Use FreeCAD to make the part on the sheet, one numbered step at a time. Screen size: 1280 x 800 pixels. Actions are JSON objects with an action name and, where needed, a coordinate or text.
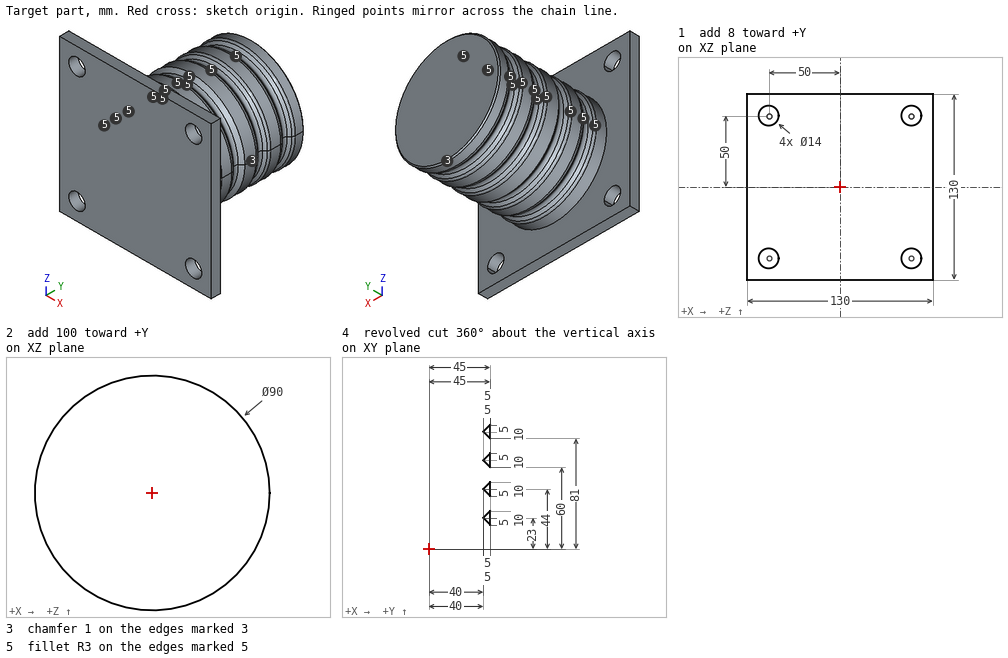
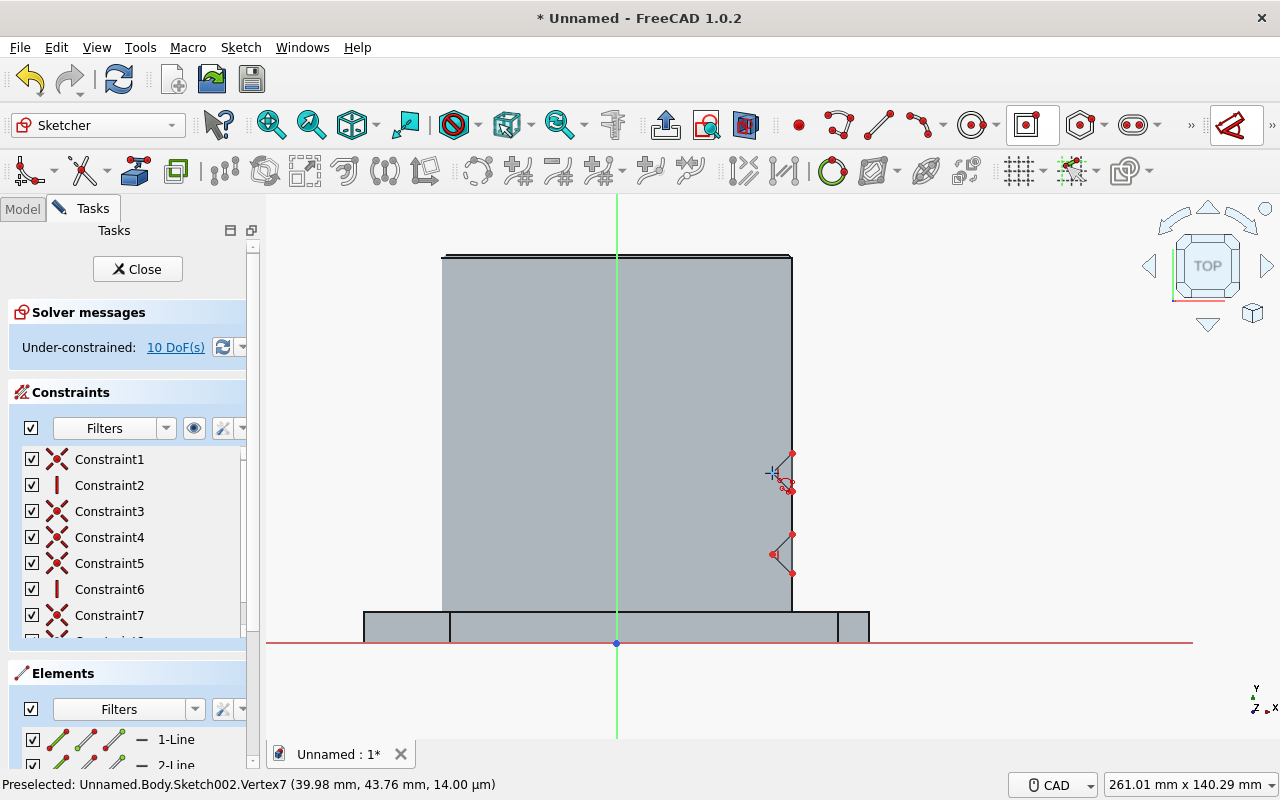
{"action": "left_click", "coordinate": [792, 410]}
{"action": "left_click", "coordinate": [792, 371]}
{"action": "left_click", "coordinate": [772, 390]}
{"action": "left_click", "coordinate": [792, 411]}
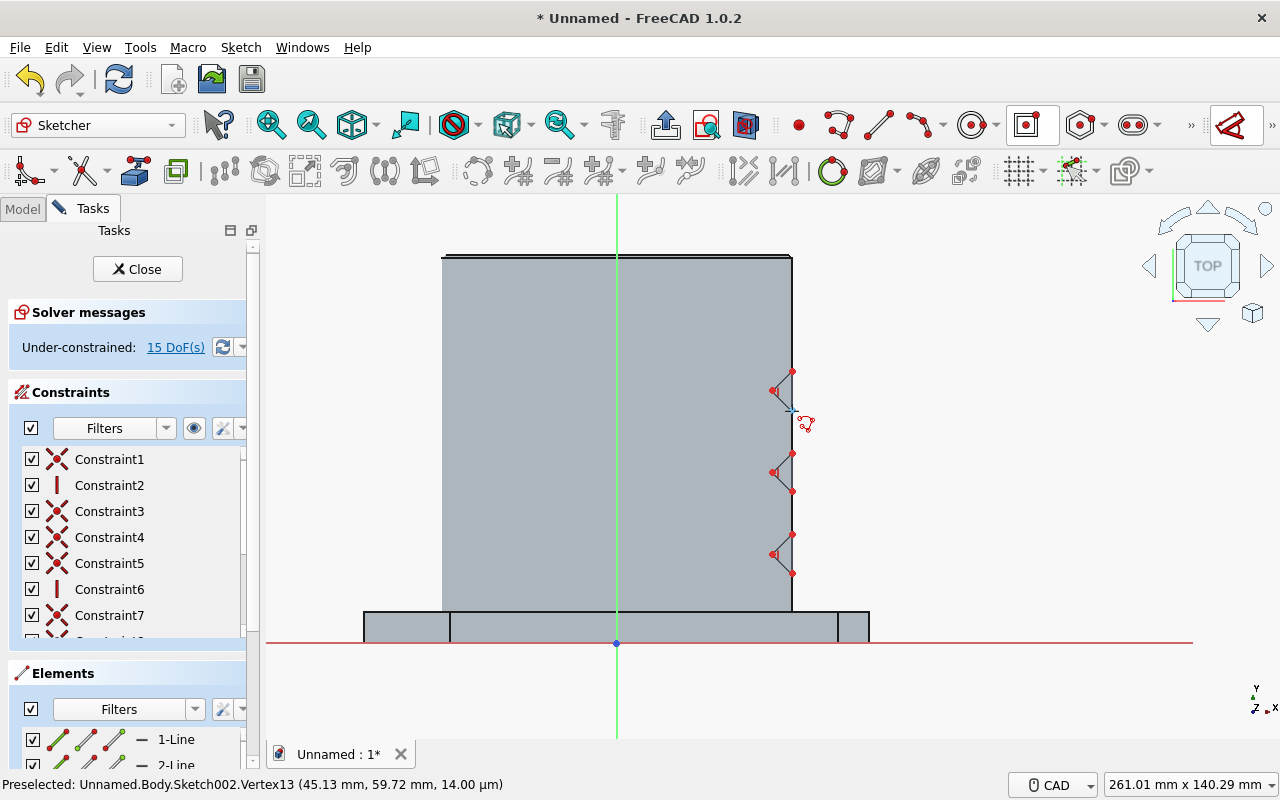
{"action": "left_click", "coordinate": [792, 328]}
{"action": "left_click", "coordinate": [792, 289]}
{"action": "left_click", "coordinate": [772, 309]}
{"action": "left_click", "coordinate": [792, 329]}
{"action": "key", "text": "Escape"}
{"action": "key", "text": "Escape"}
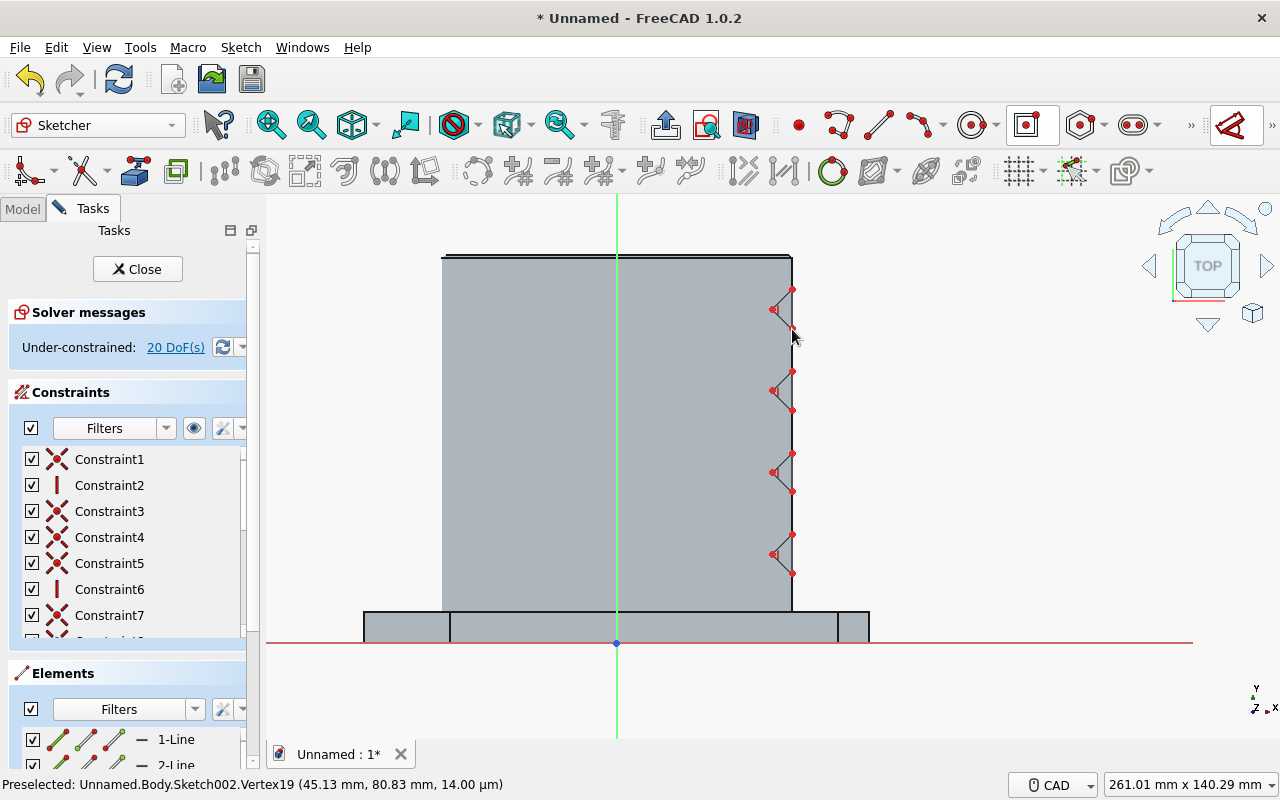
{"action": "left_click", "coordinate": [792, 558]}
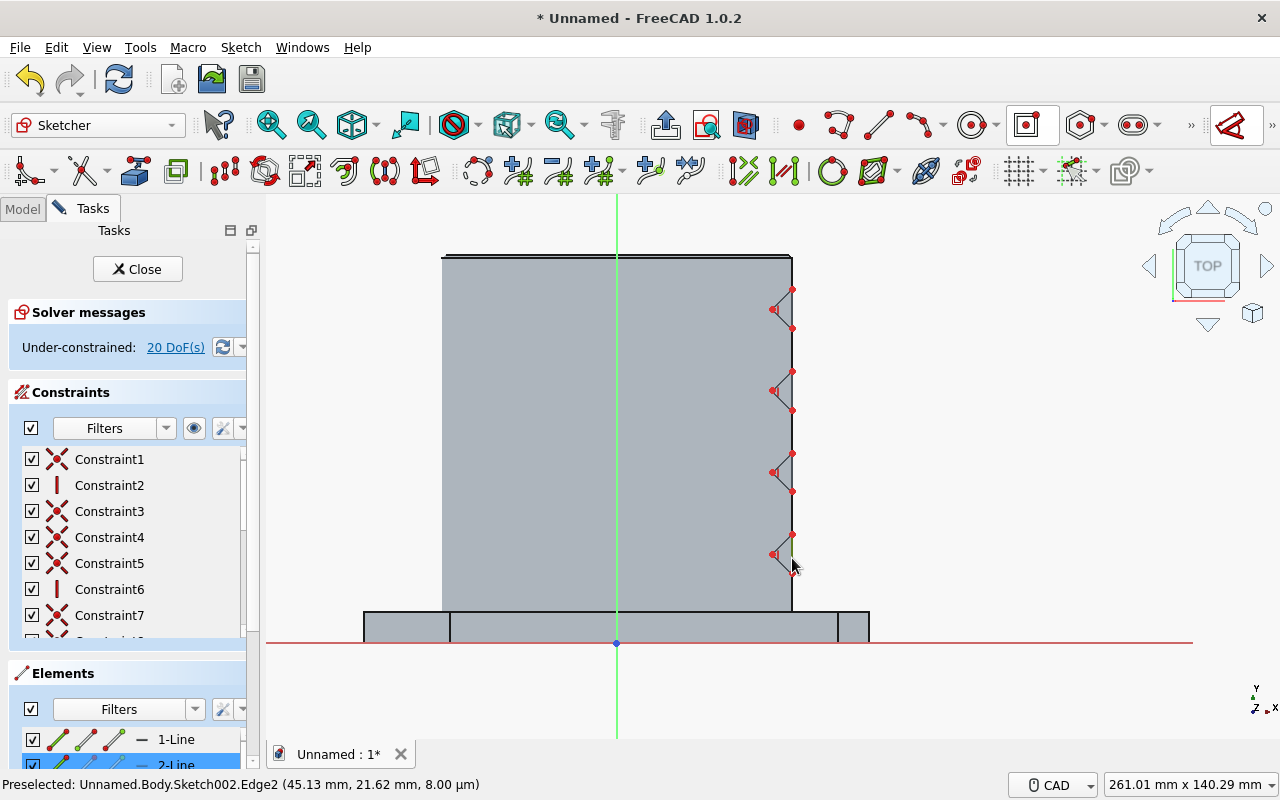
{"action": "key", "text": "i"}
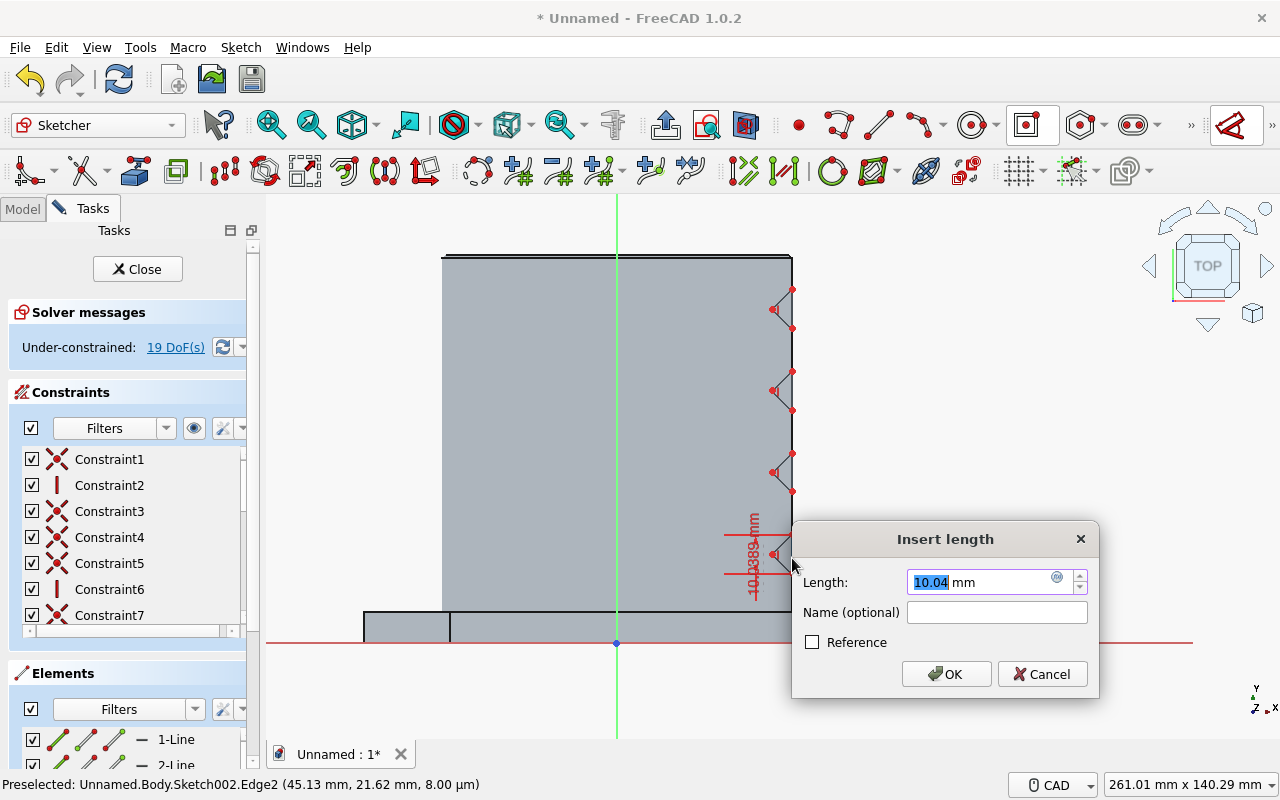
{"action": "type", "text": "10"}
{"action": "key", "text": "Return"}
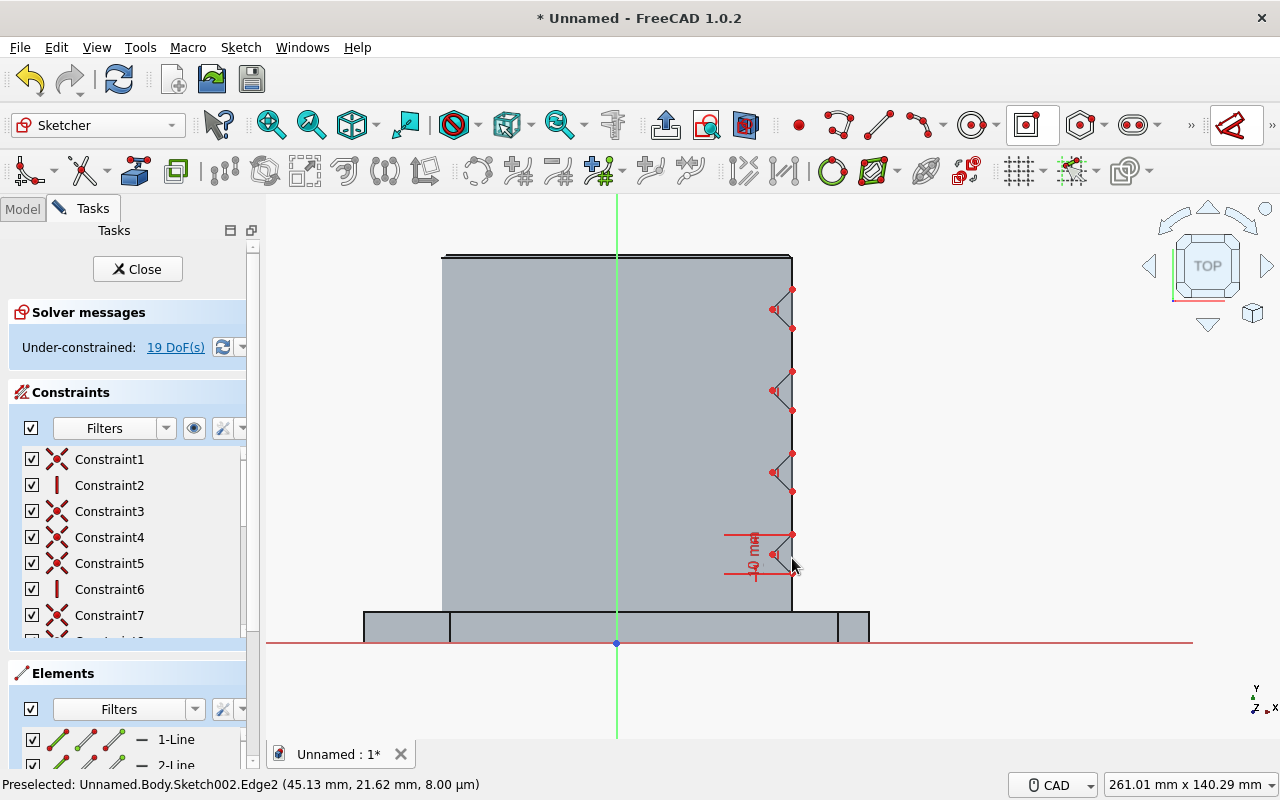
{"action": "scroll", "coordinate": [792, 477], "scroll_direction": "up", "scroll_amount": 2}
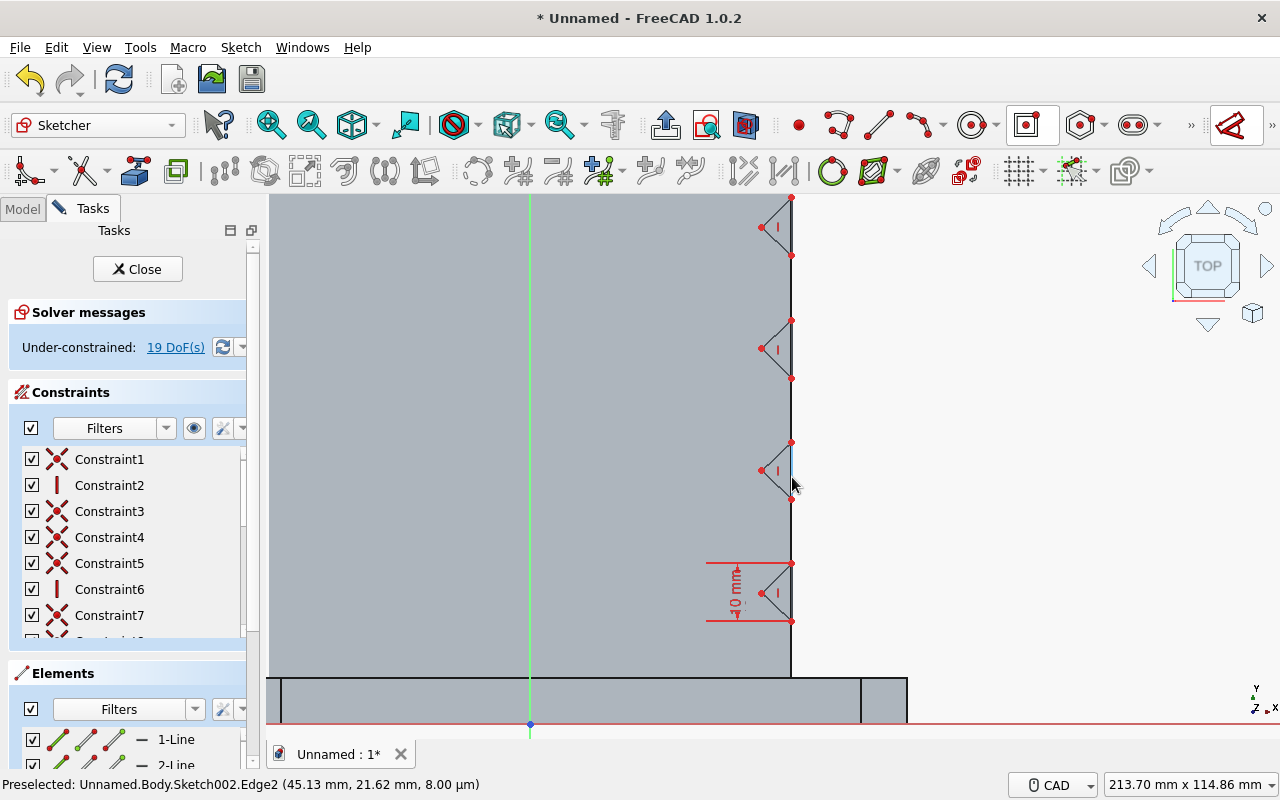
{"action": "left_click", "coordinate": [792, 476]}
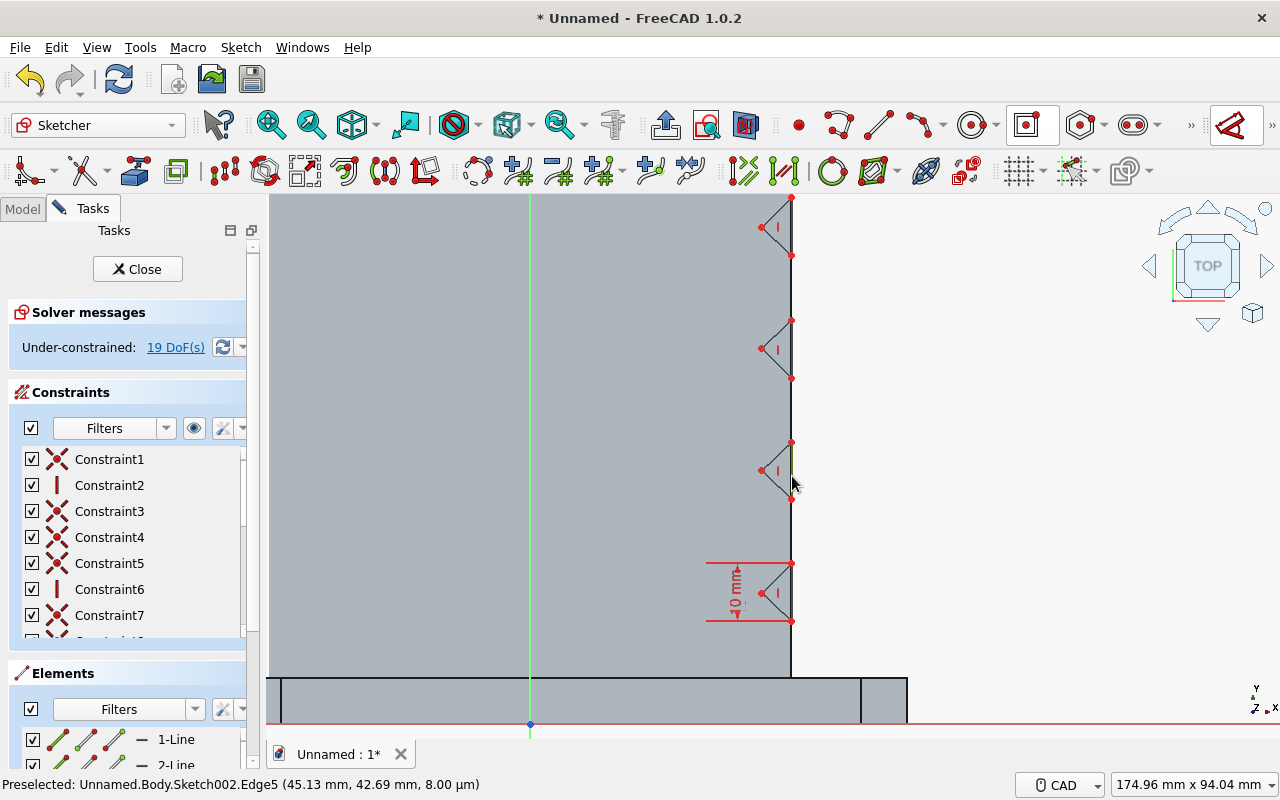
{"action": "key", "text": "i"}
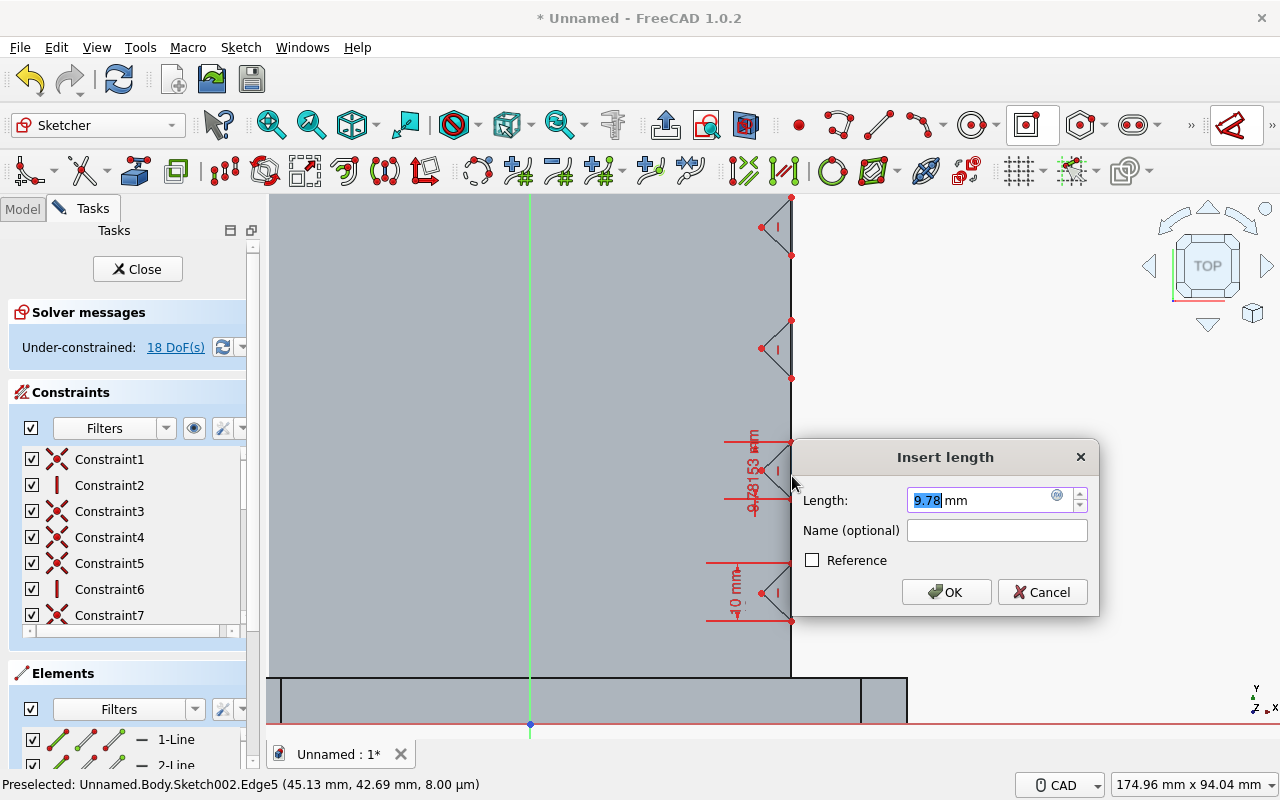
{"action": "type", "text": "10"}
{"action": "key", "text": "Return"}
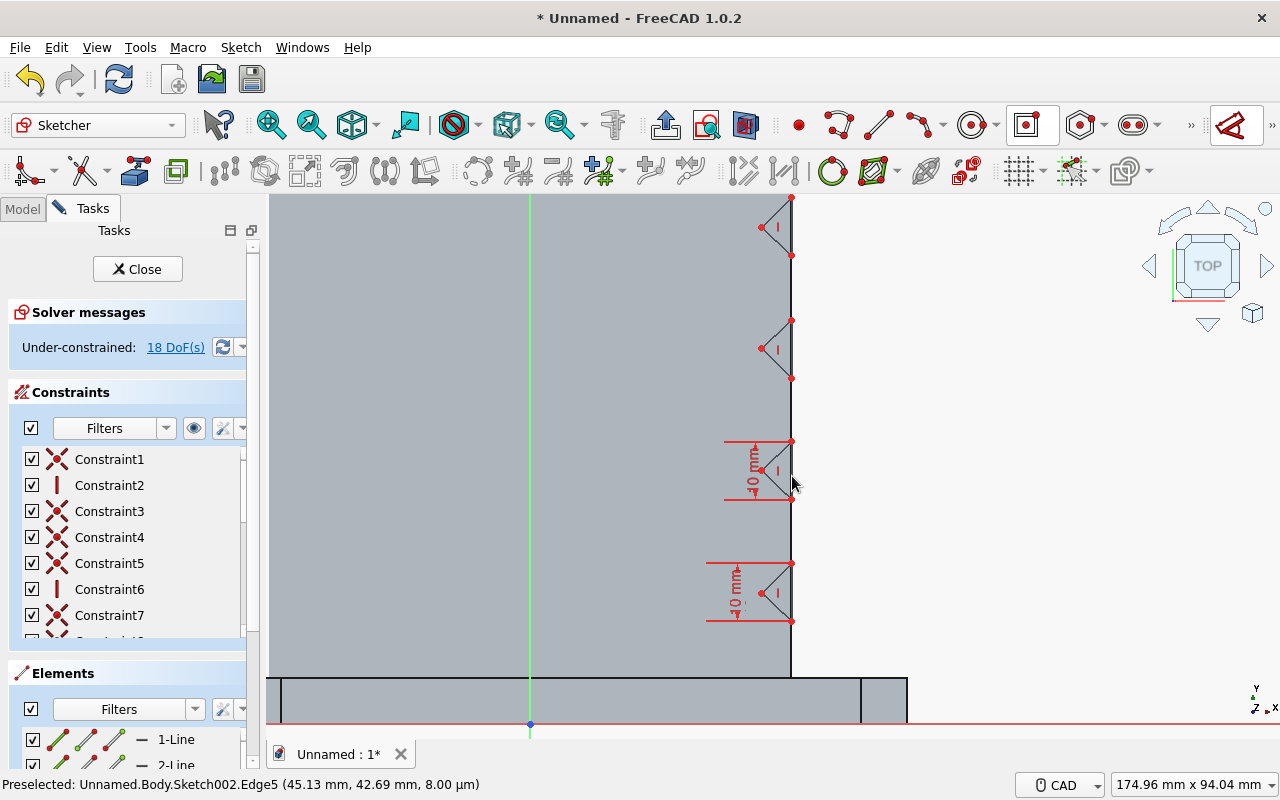
{"action": "left_click", "coordinate": [792, 361]}